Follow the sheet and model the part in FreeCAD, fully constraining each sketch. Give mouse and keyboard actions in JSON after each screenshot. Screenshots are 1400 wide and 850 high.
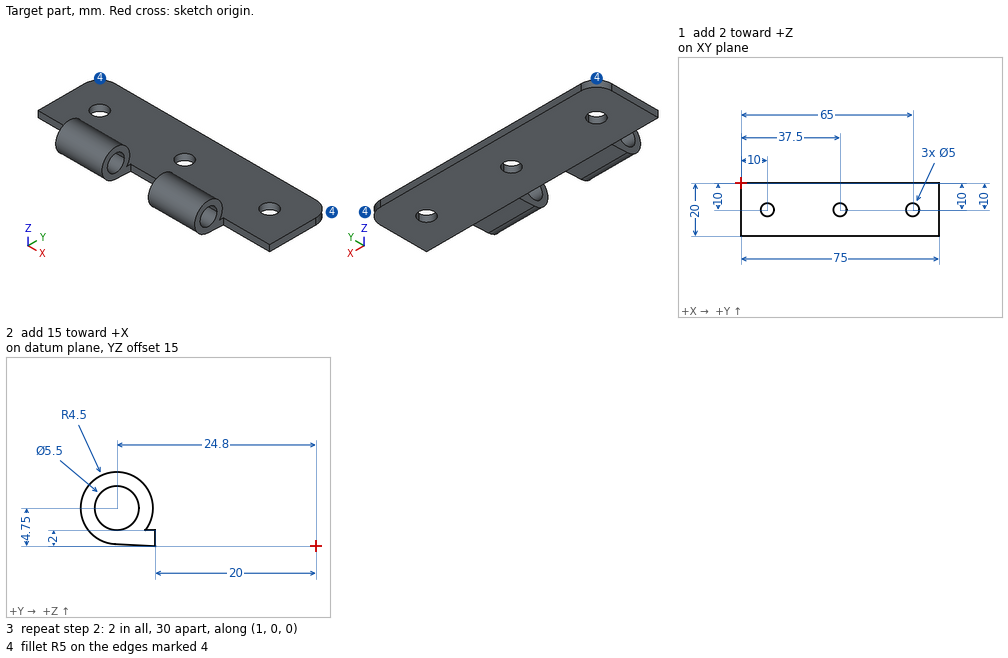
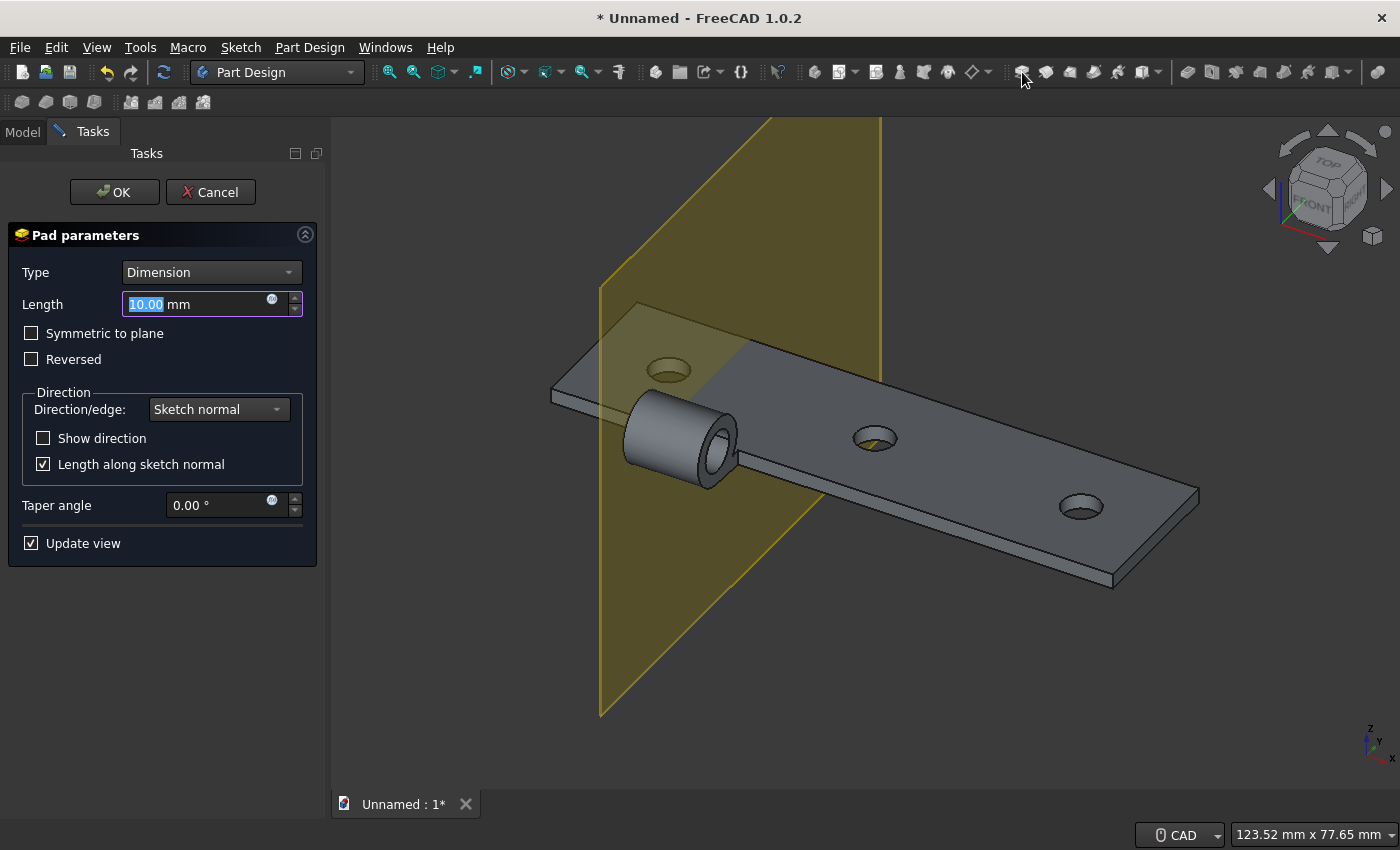
{"action": "type", "text": "15"}
{"action": "key", "text": "Tab"}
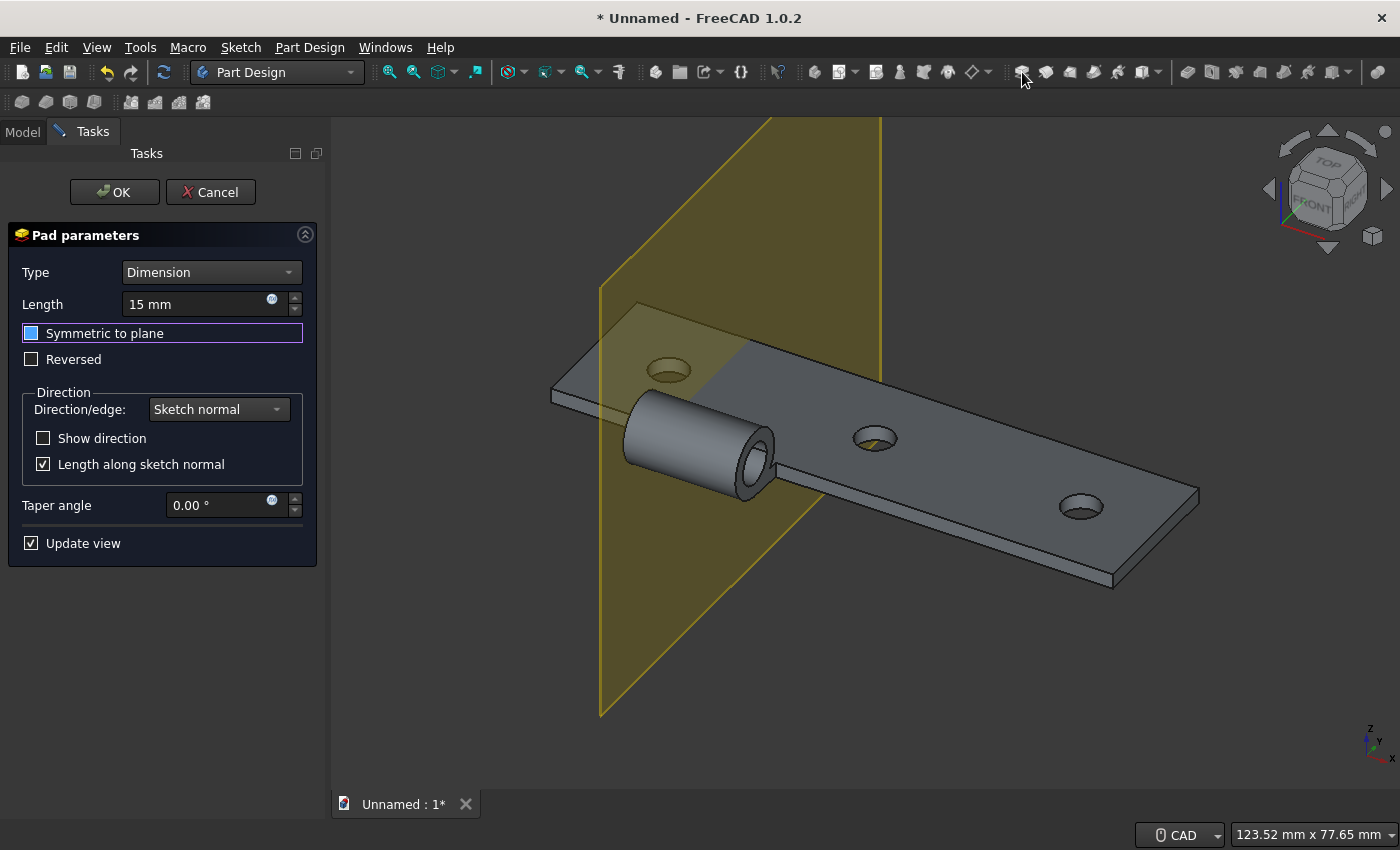
{"action": "left_click", "coordinate": [115, 192]}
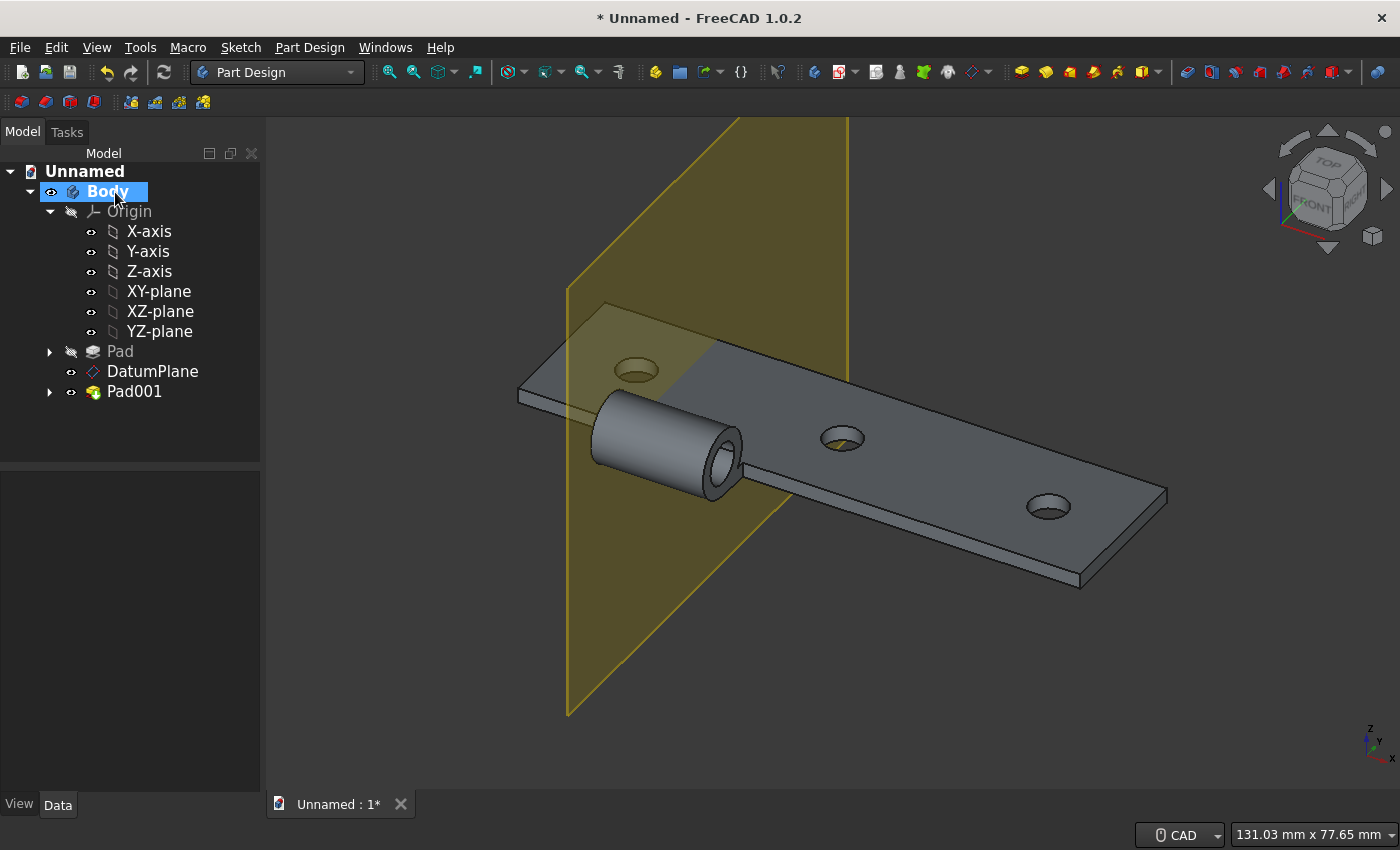
{"action": "left_click", "coordinate": [116, 372]}
{"action": "key", "text": "space"}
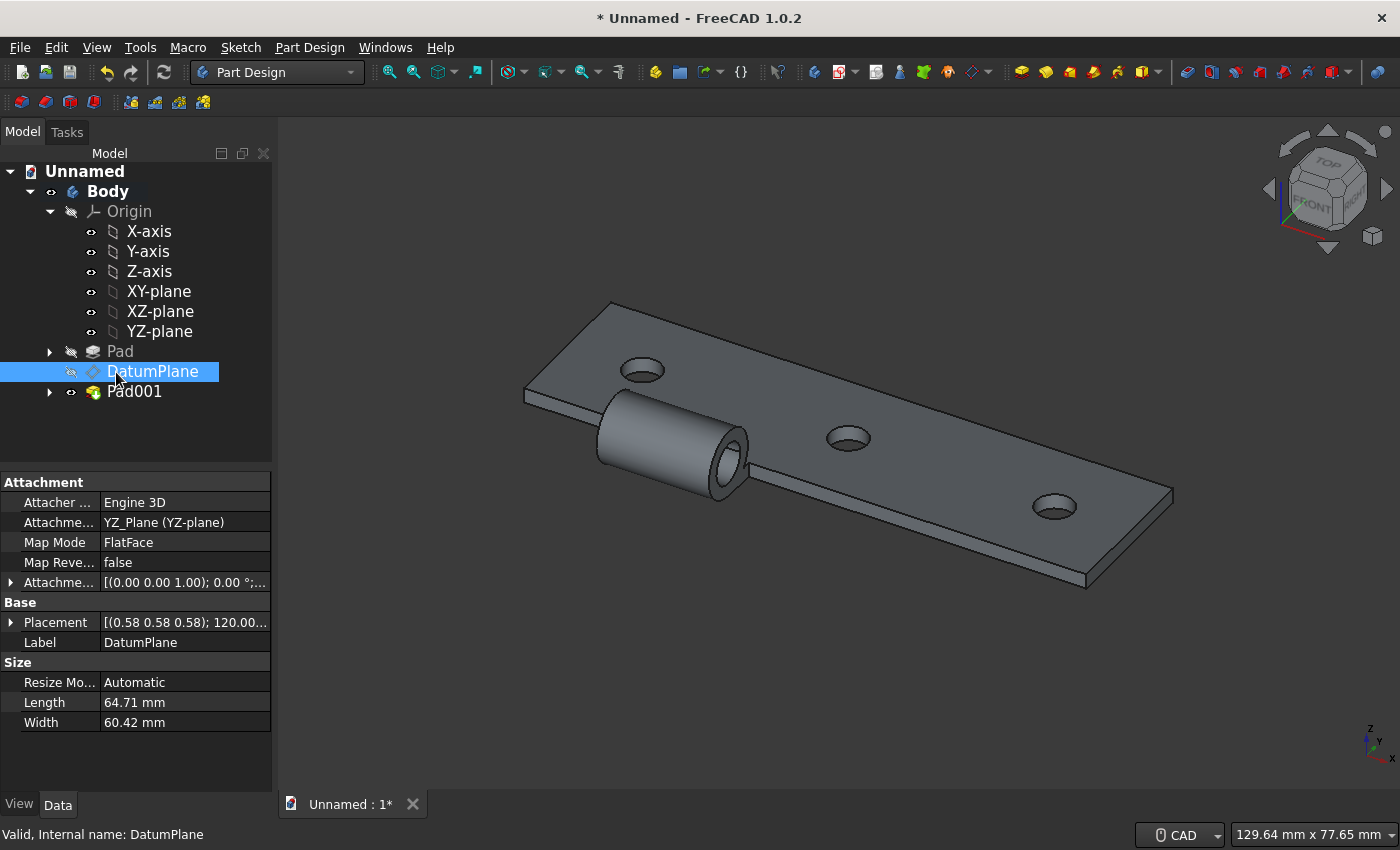
{"action": "left_click", "coordinate": [116, 392]}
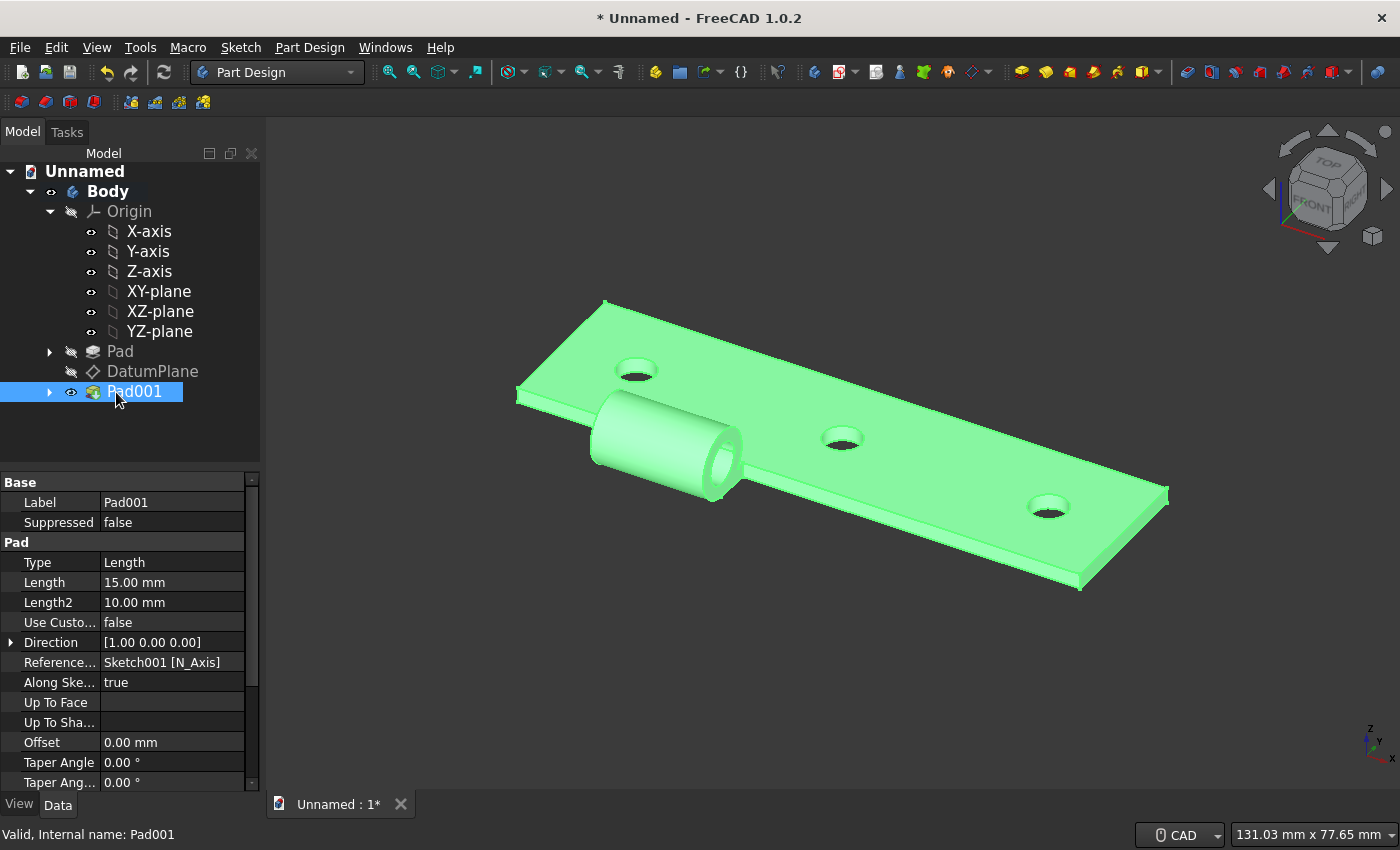
{"action": "left_click", "coordinate": [156, 102]}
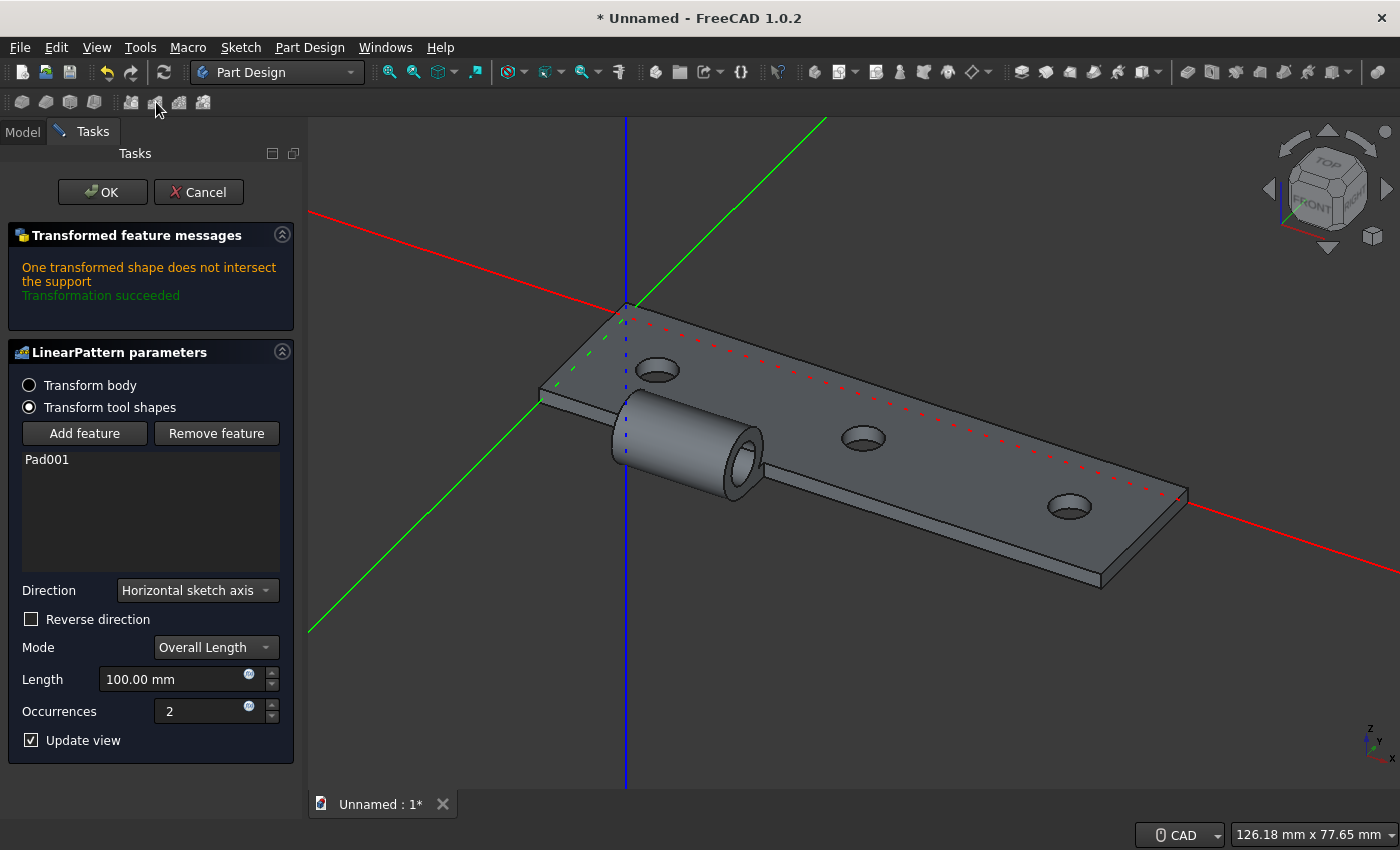
{"action": "left_click", "coordinate": [198, 590]}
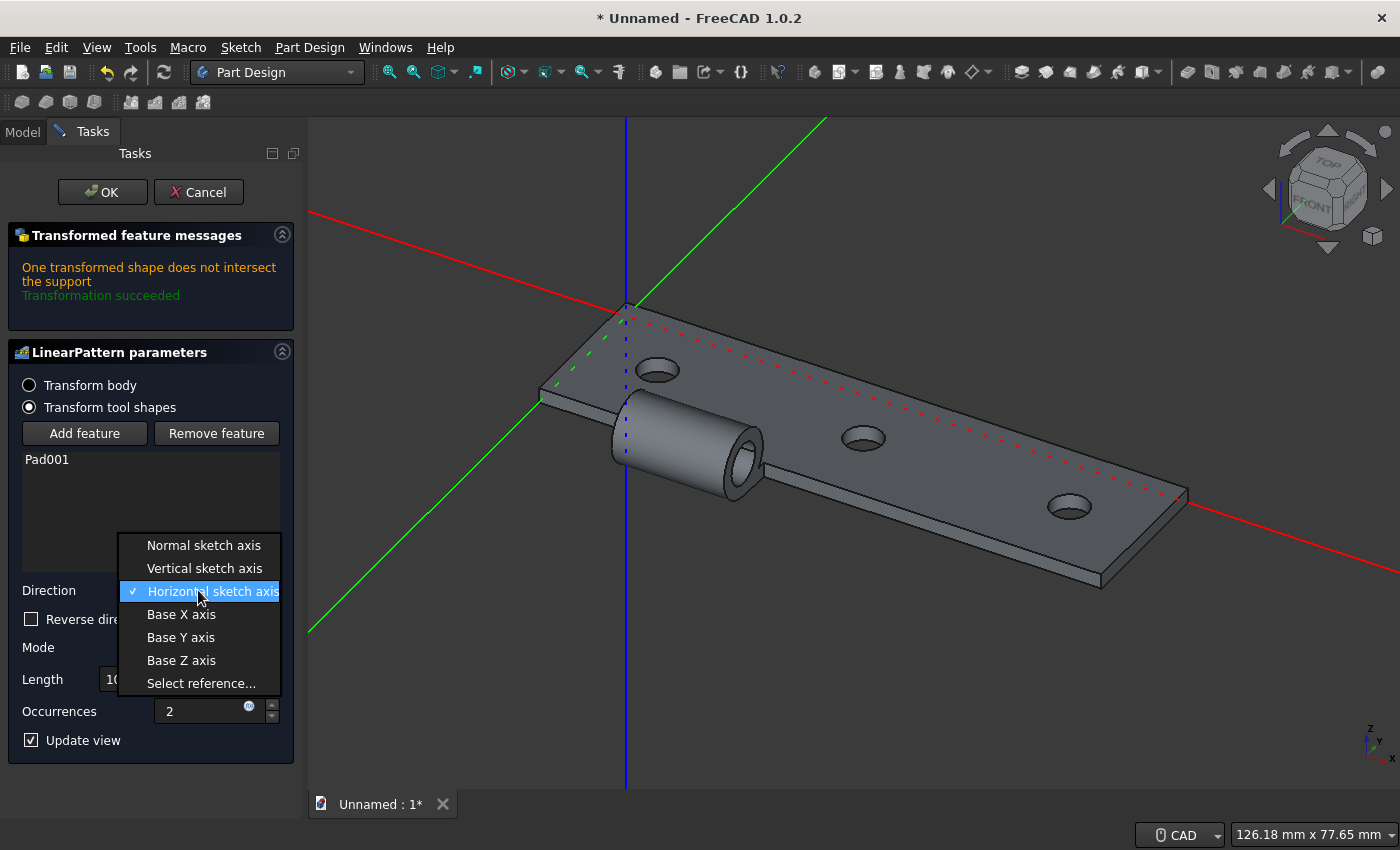
{"action": "left_click", "coordinate": [198, 614]}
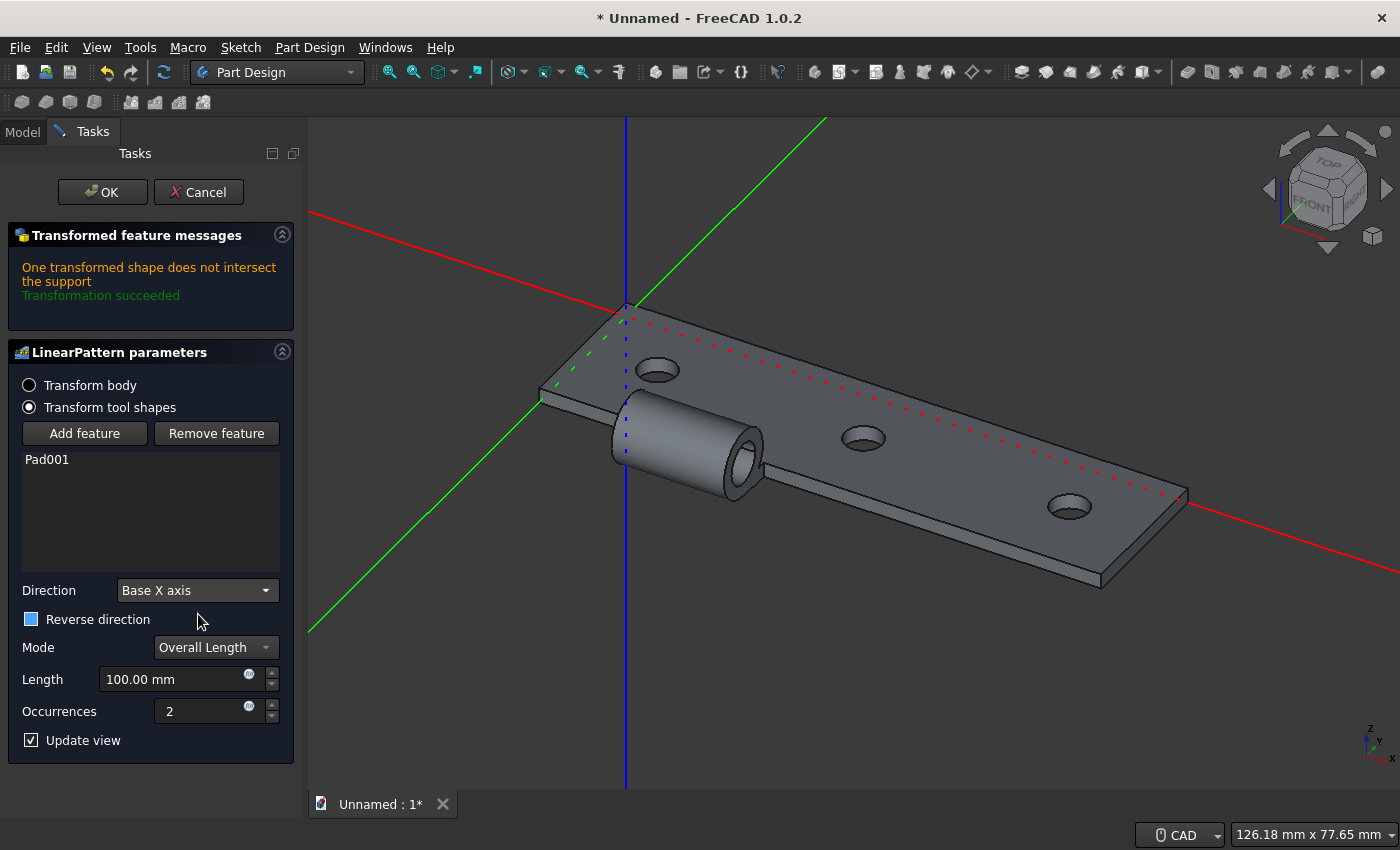
{"action": "left_click", "coordinate": [217, 648]}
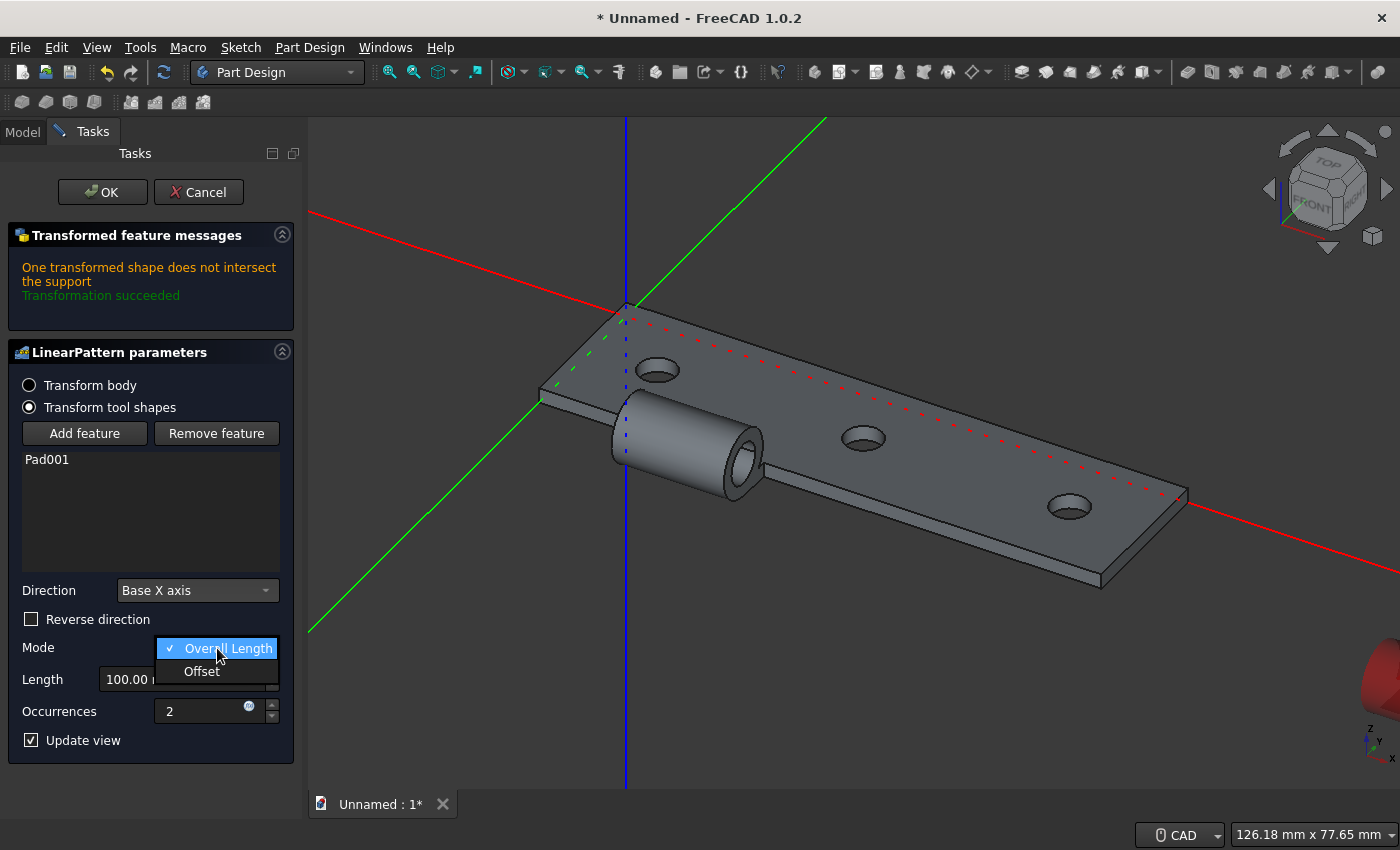
{"action": "left_click", "coordinate": [216, 672]}